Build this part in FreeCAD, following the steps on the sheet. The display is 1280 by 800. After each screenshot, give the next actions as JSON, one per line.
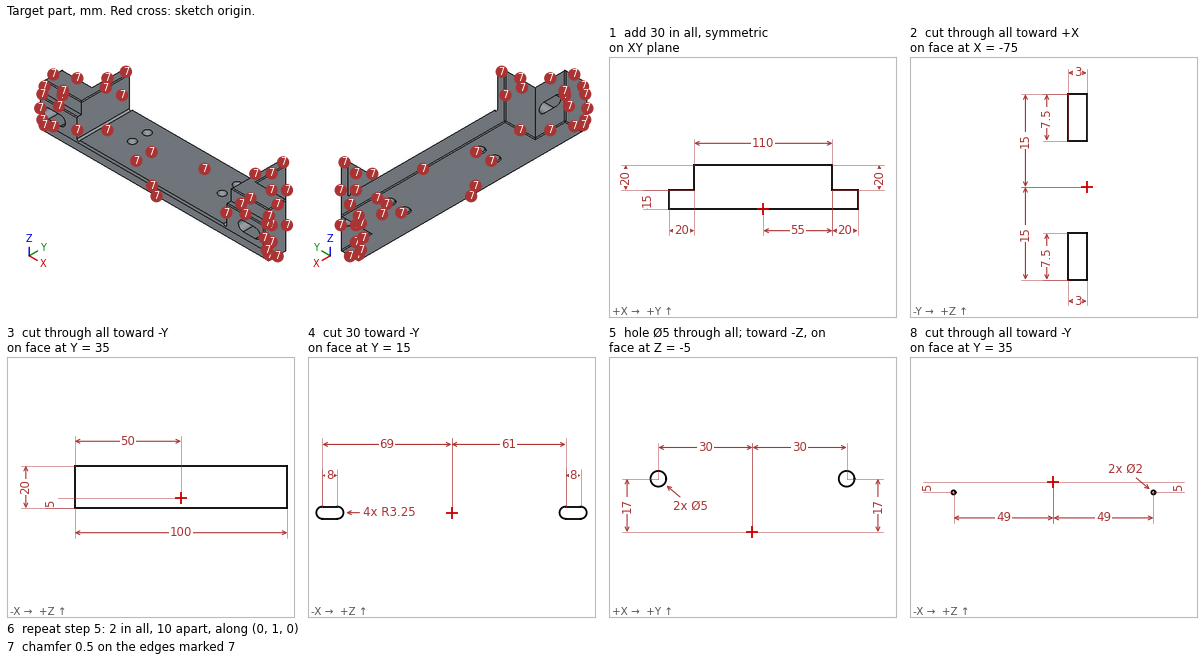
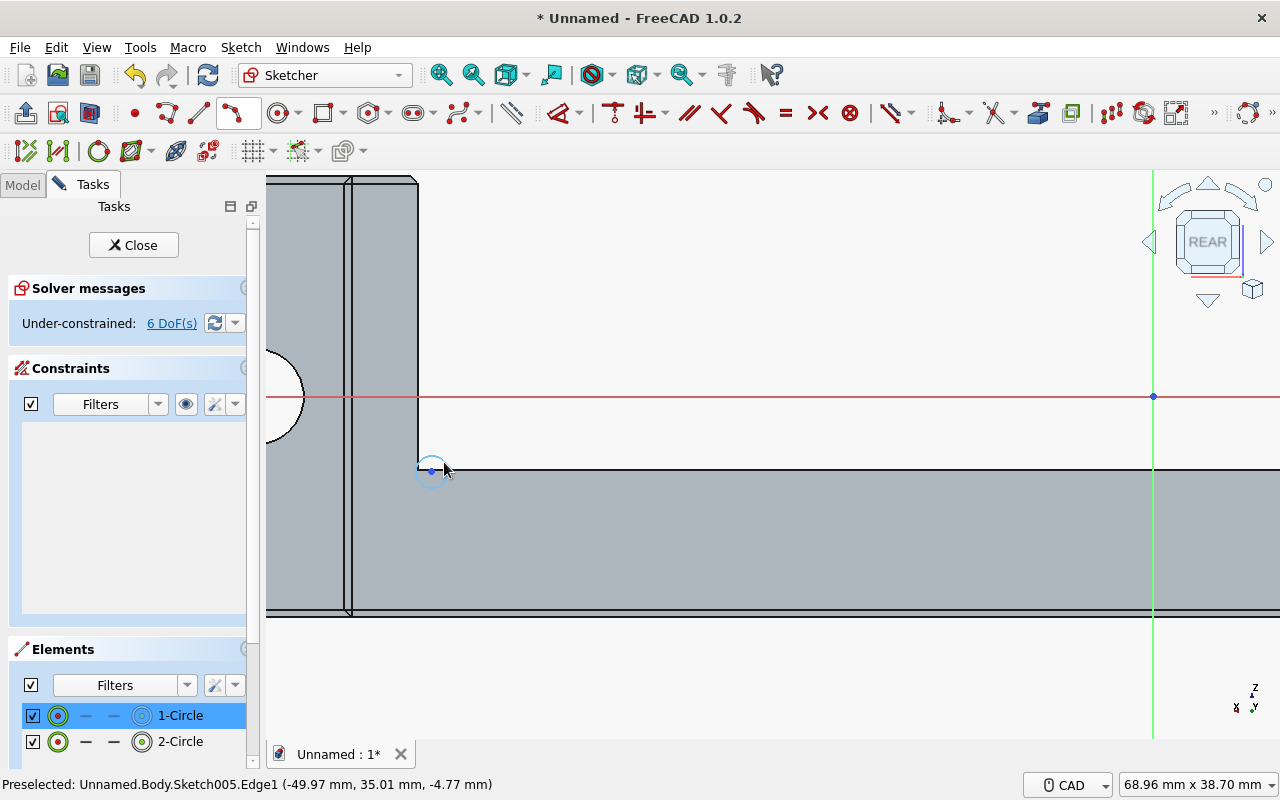
{"action": "left_click", "coordinate": [443, 461]}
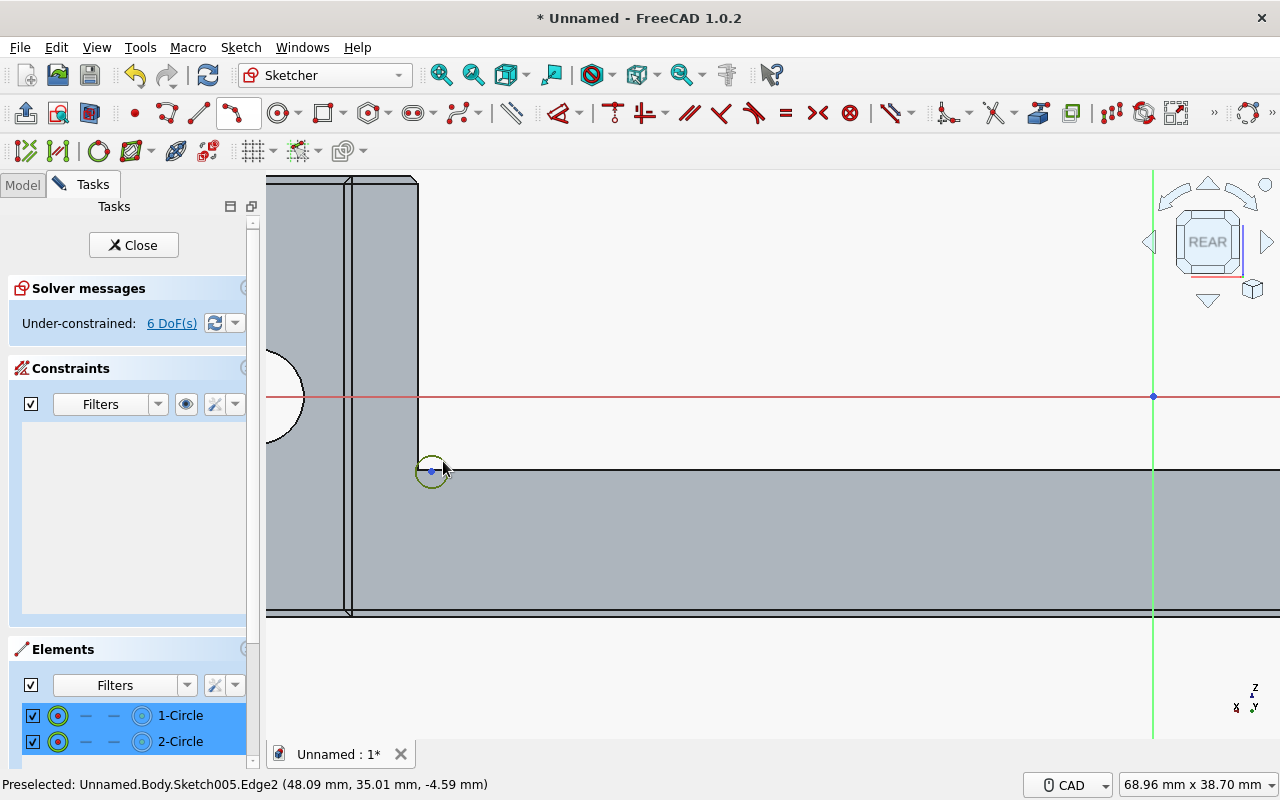
{"action": "left_click", "coordinate": [786, 114]}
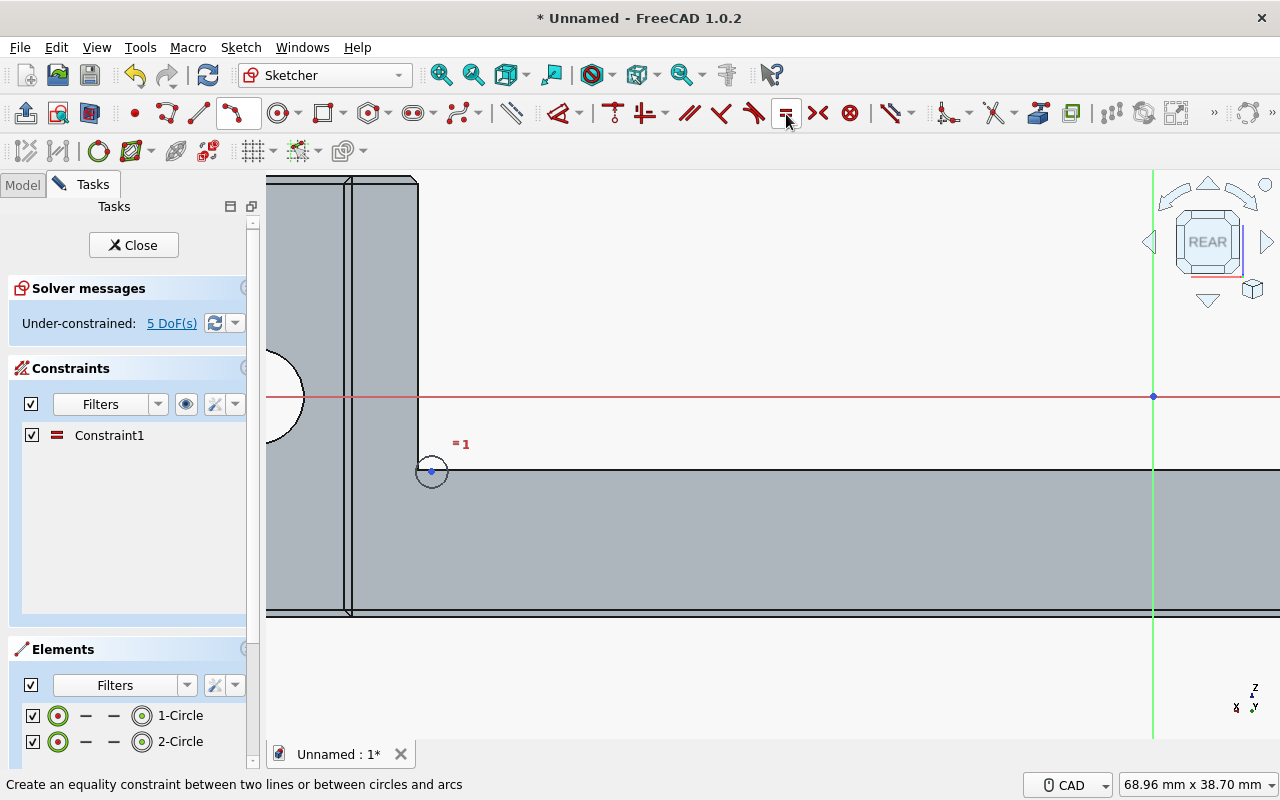
{"action": "left_click", "coordinate": [558, 114]}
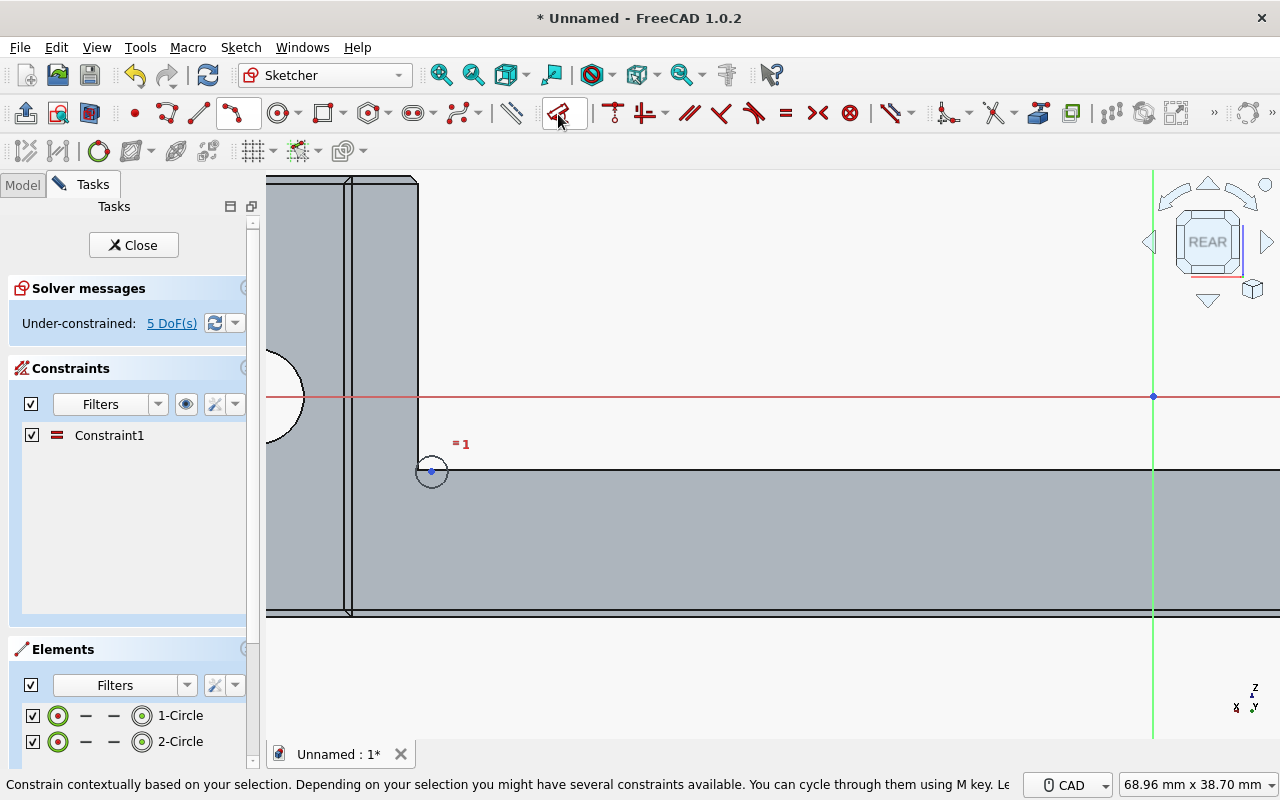
{"action": "scroll", "coordinate": [443, 462], "scroll_direction": "down", "scroll_amount": 5}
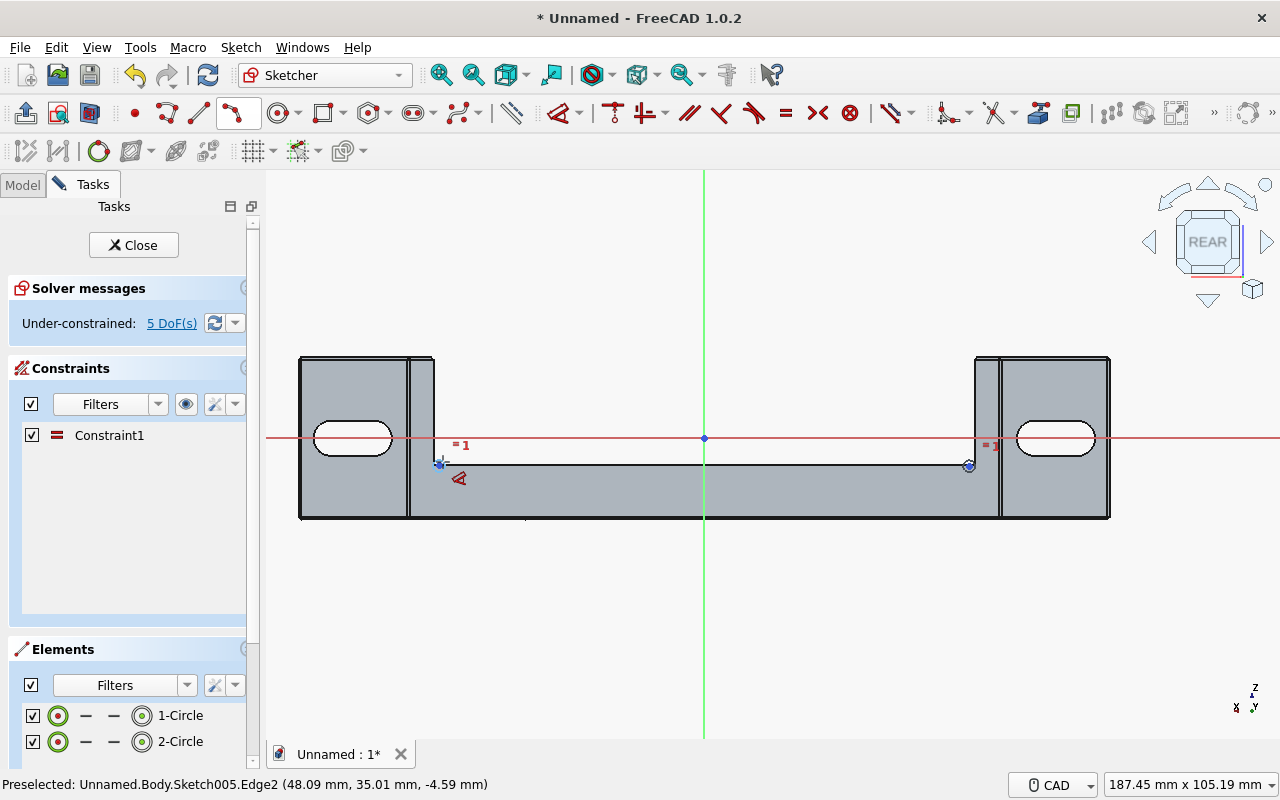
{"action": "scroll", "coordinate": [973, 462], "scroll_direction": "up", "scroll_amount": 7}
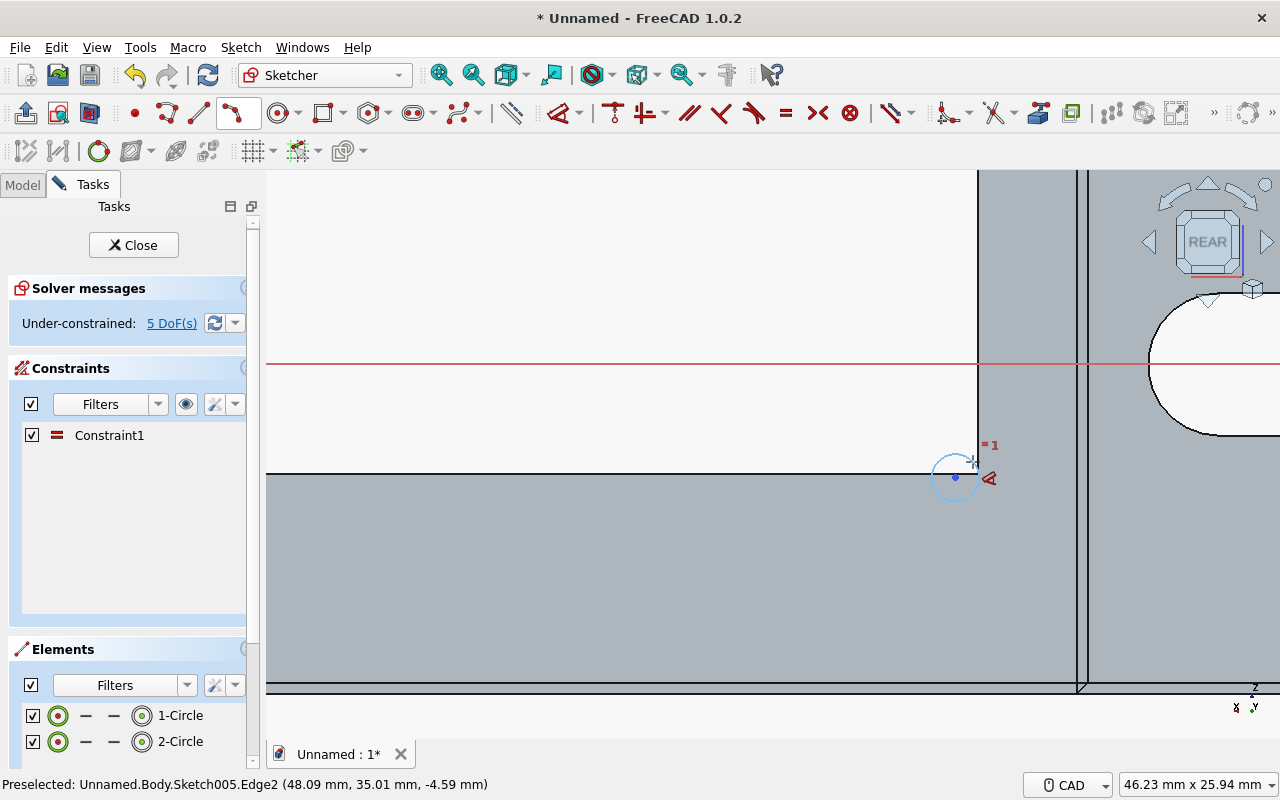
{"action": "left_click", "coordinate": [972, 461]}
{"action": "left_click", "coordinate": [994, 438]}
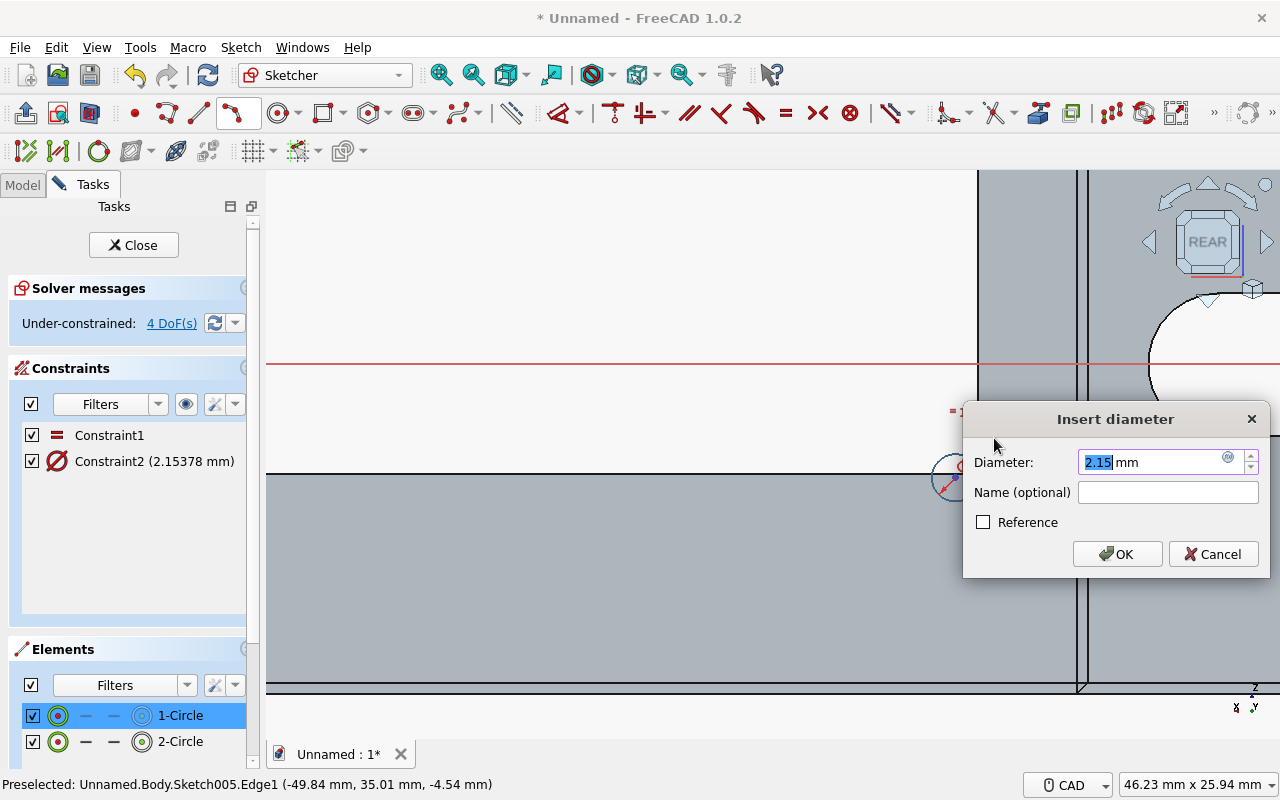
{"action": "type", "text": "2"}
{"action": "key", "text": "Return"}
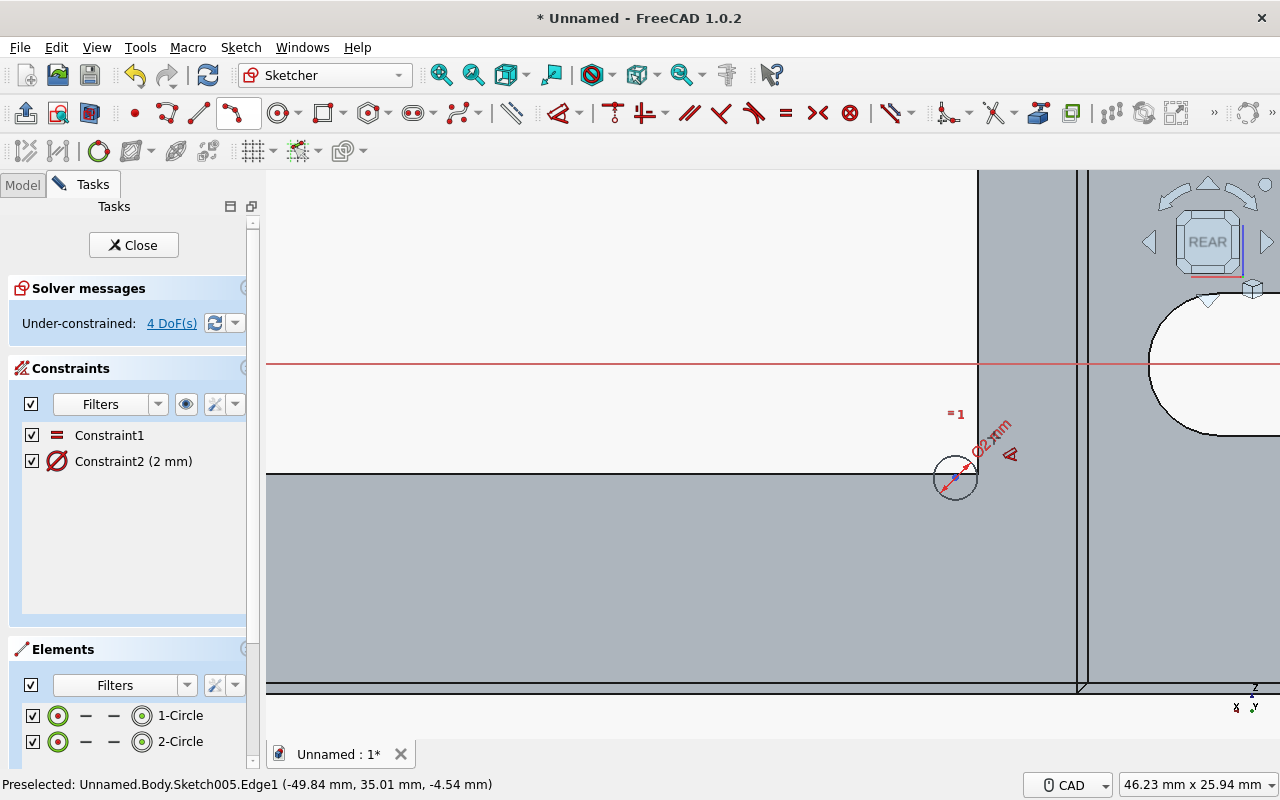
{"action": "left_click", "coordinate": [955, 478]}
{"action": "left_click", "coordinate": [989, 395]}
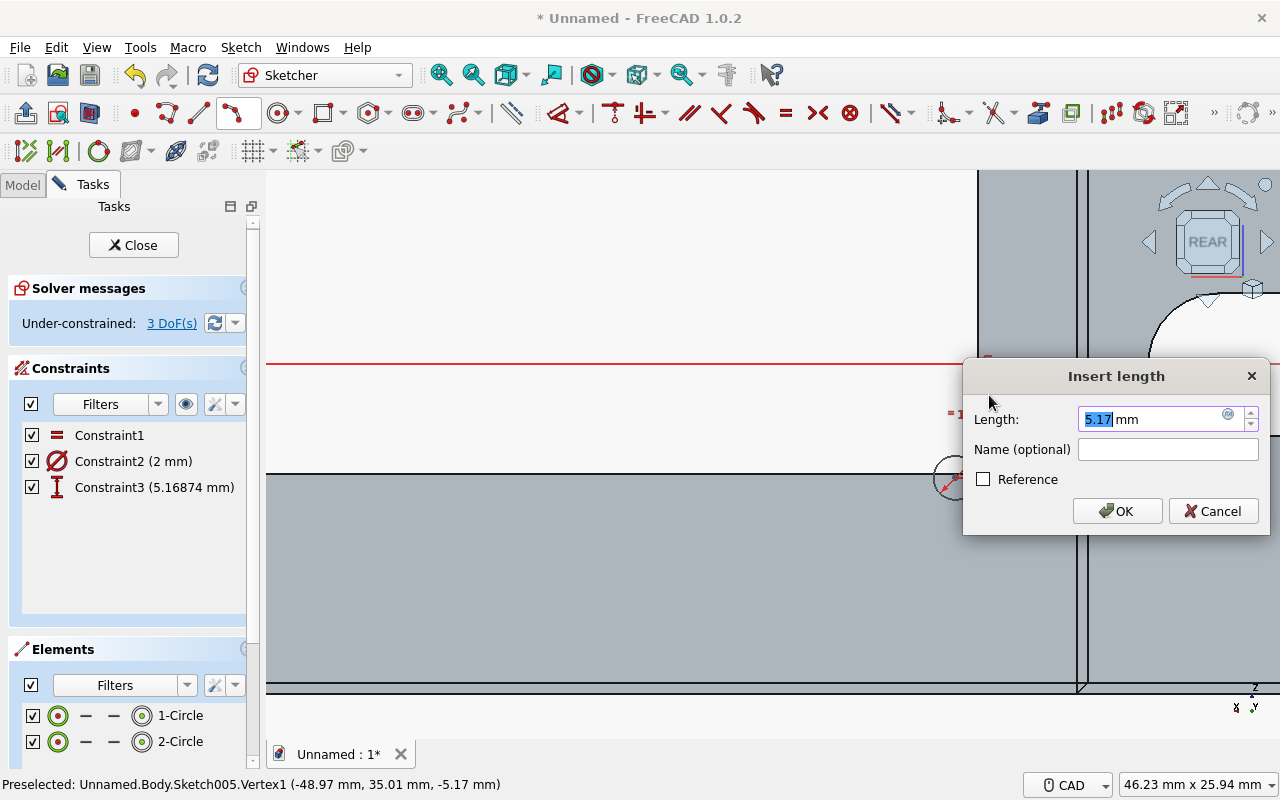
{"action": "type", "text": "5"}
{"action": "key", "text": "Return"}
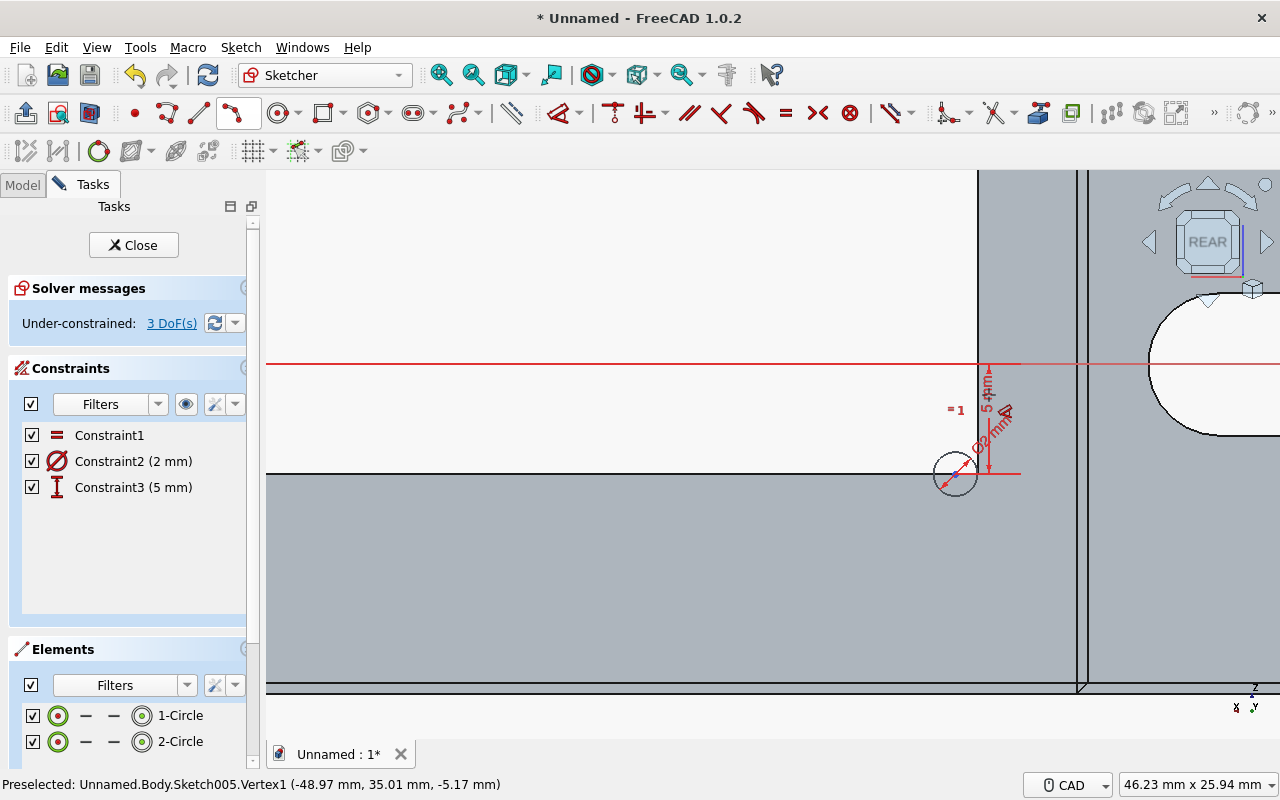
{"action": "scroll", "coordinate": [974, 462], "scroll_direction": "down", "scroll_amount": 7}